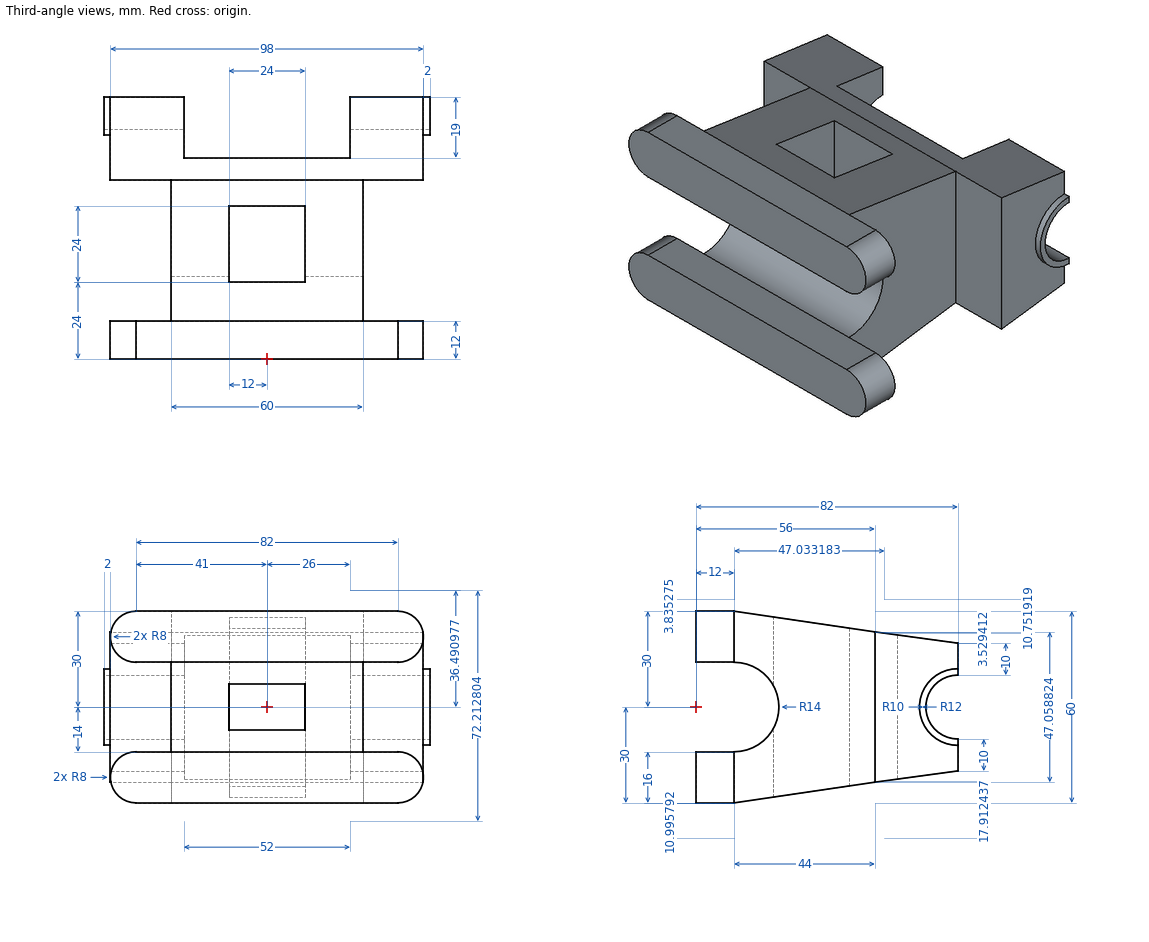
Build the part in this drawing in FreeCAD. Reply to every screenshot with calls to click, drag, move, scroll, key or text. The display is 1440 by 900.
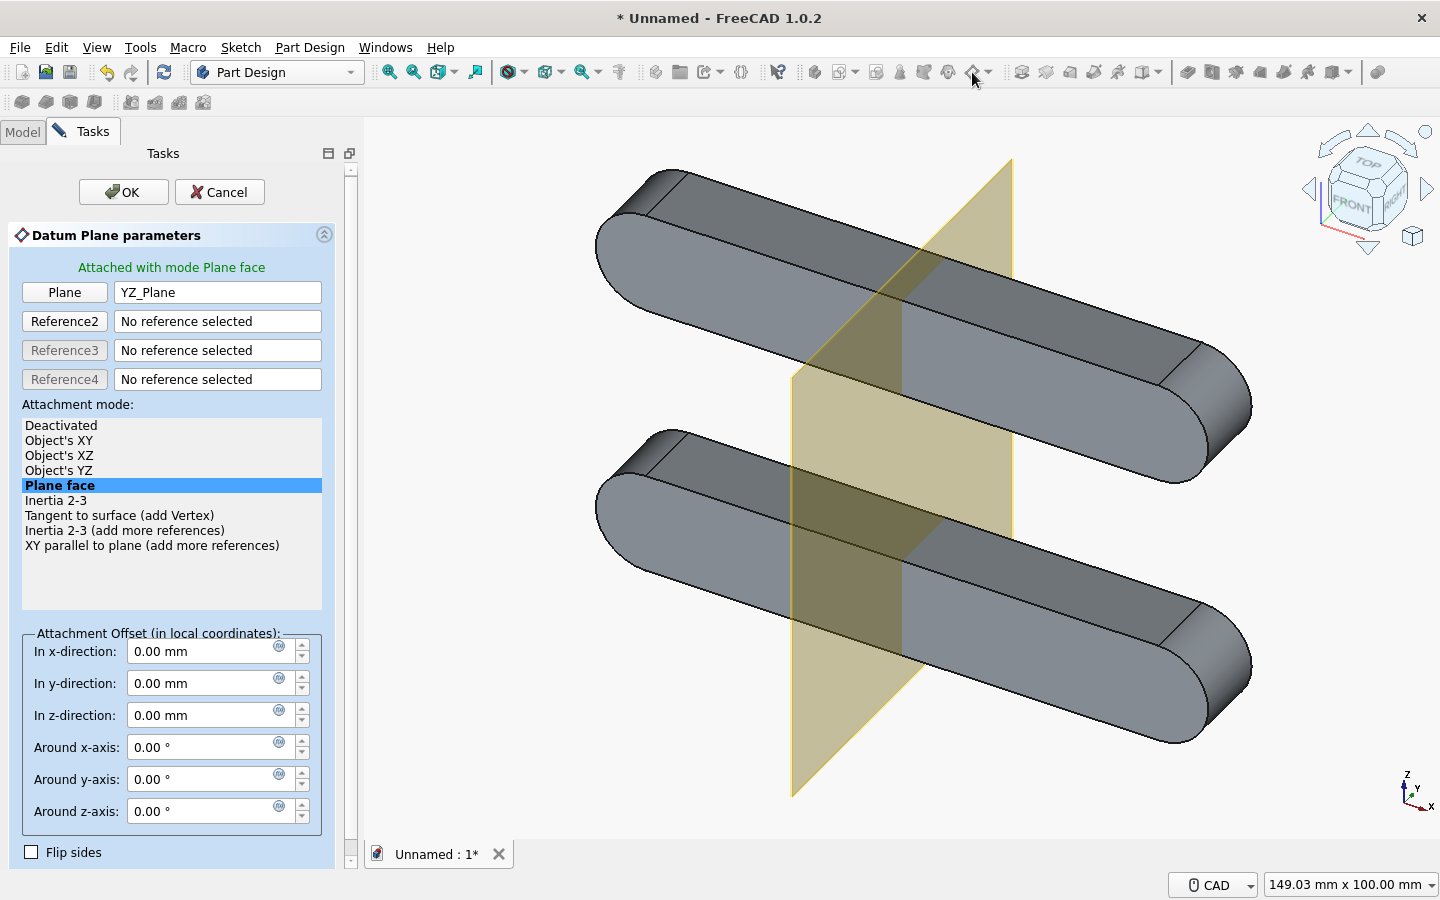
triple_click(210, 715)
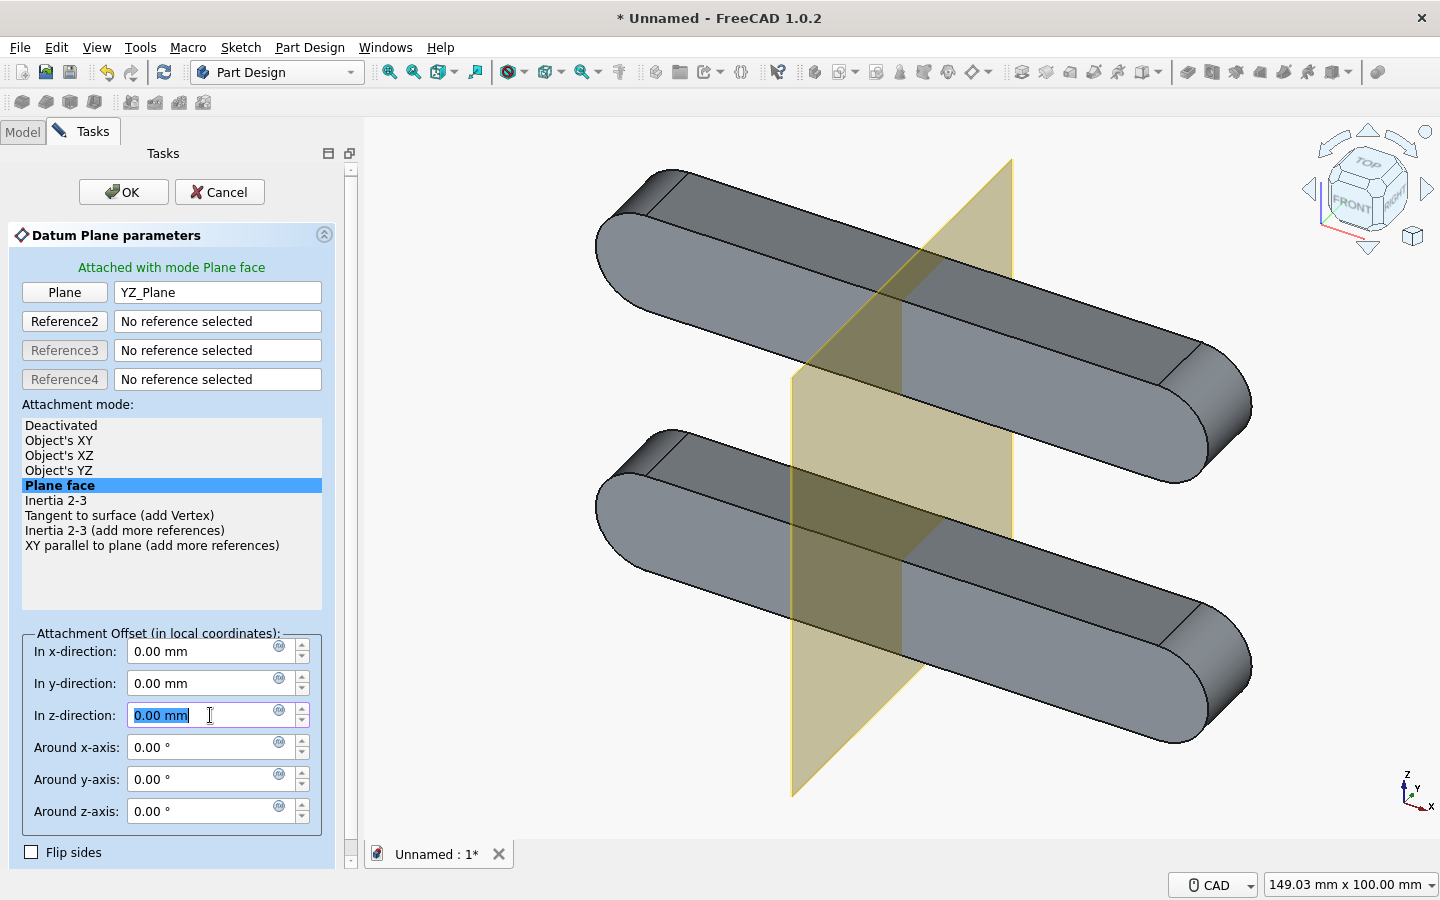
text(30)
key(Tab)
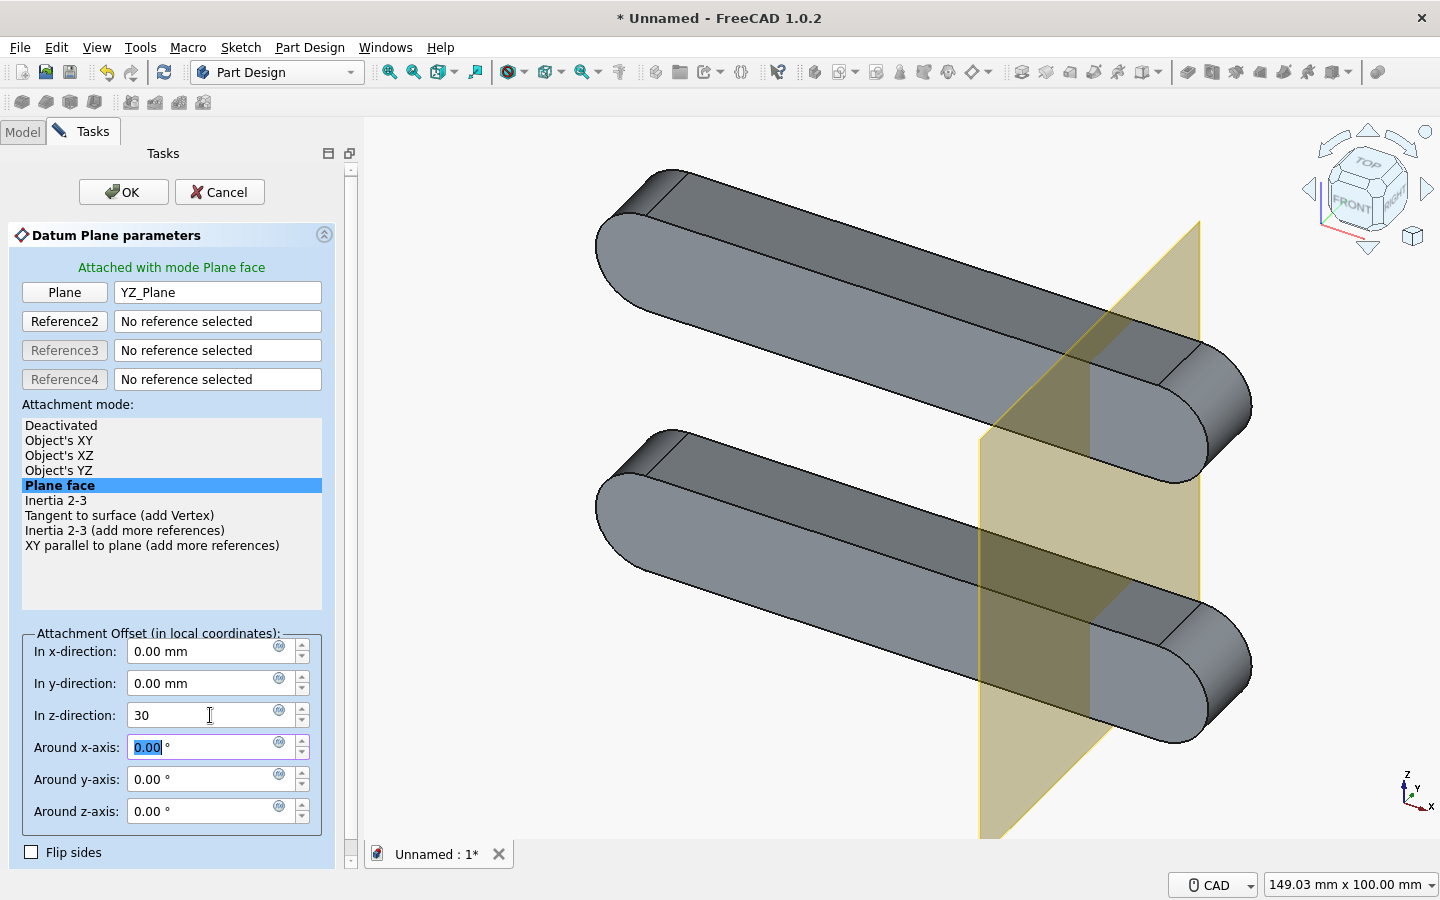
click(124, 192)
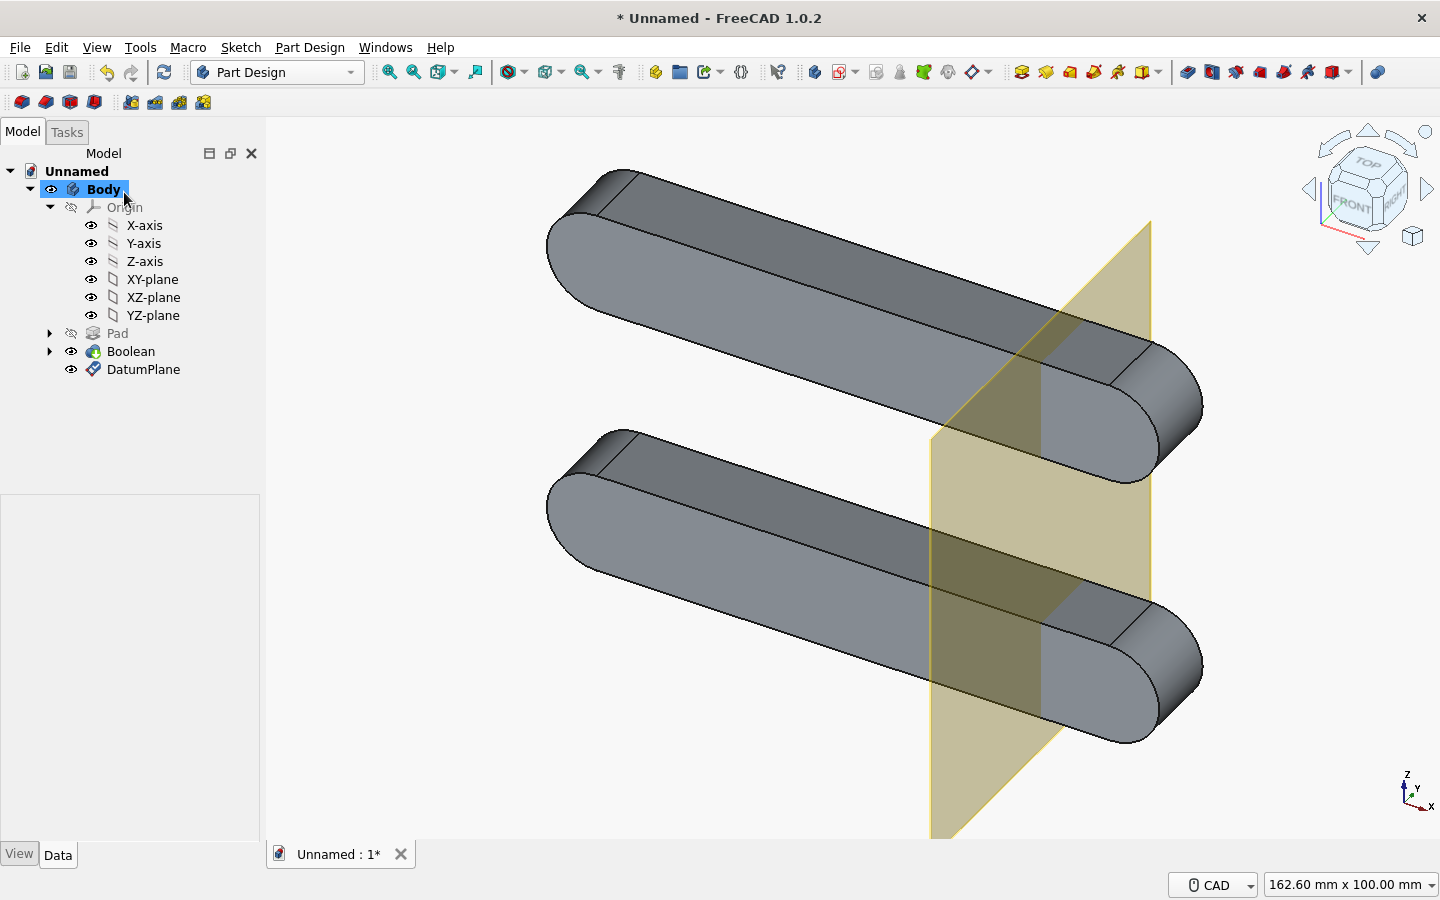
click(116, 369)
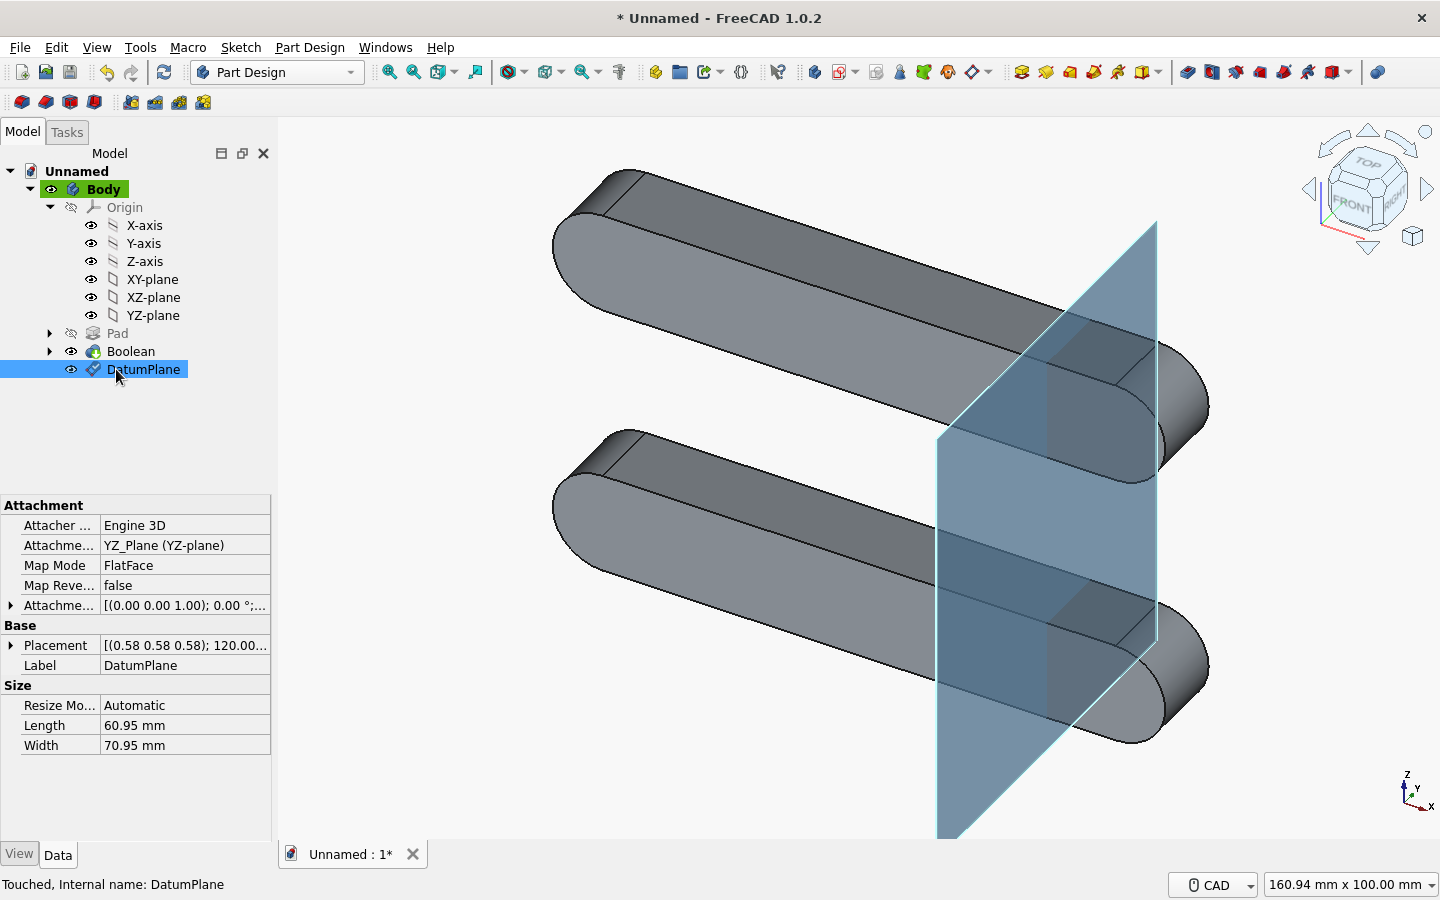
click(840, 72)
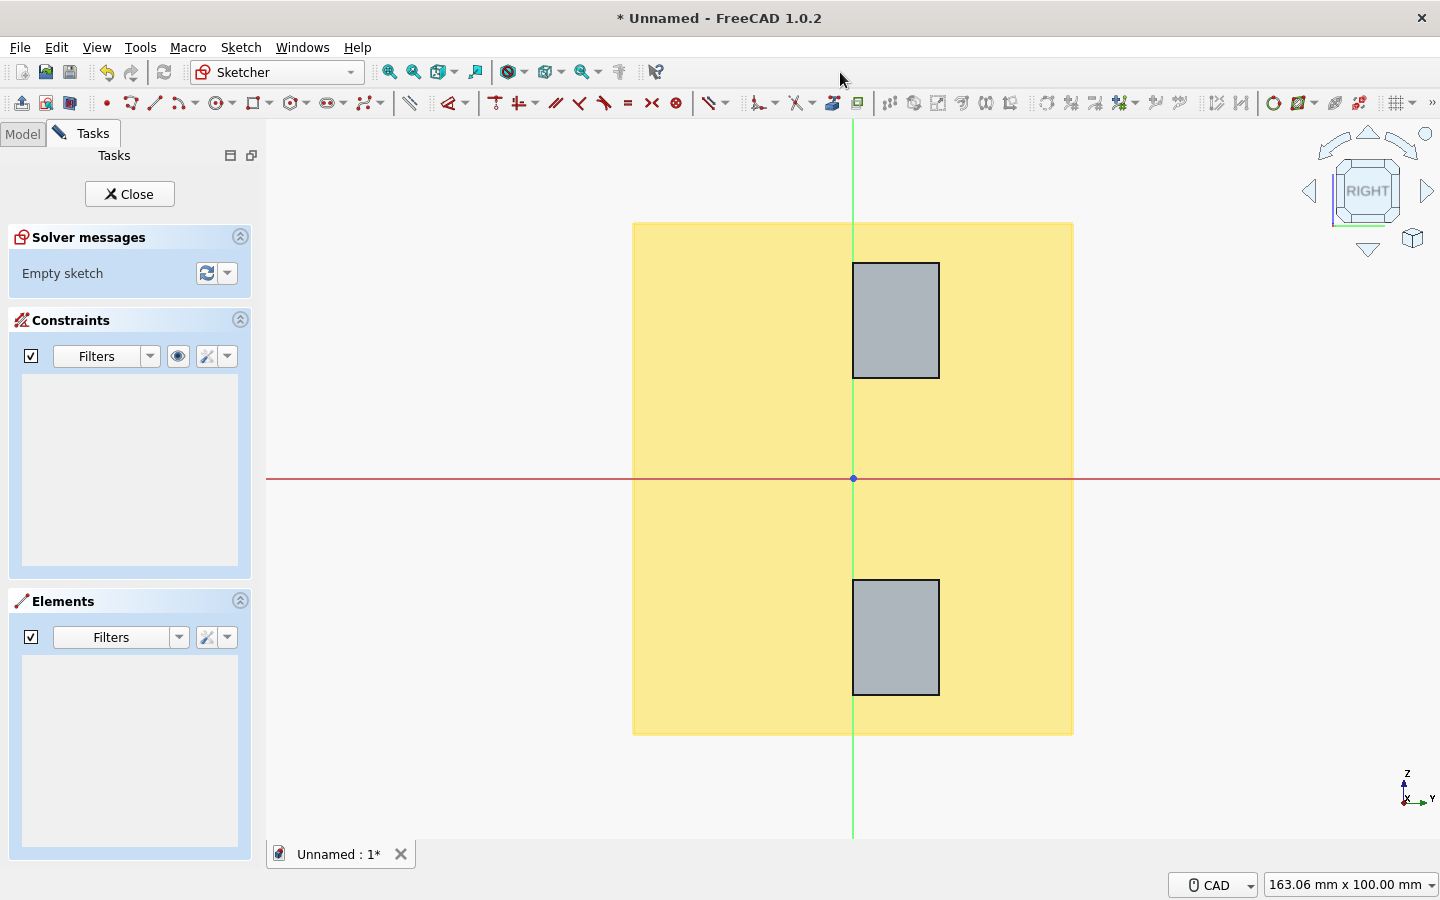
click(70, 104)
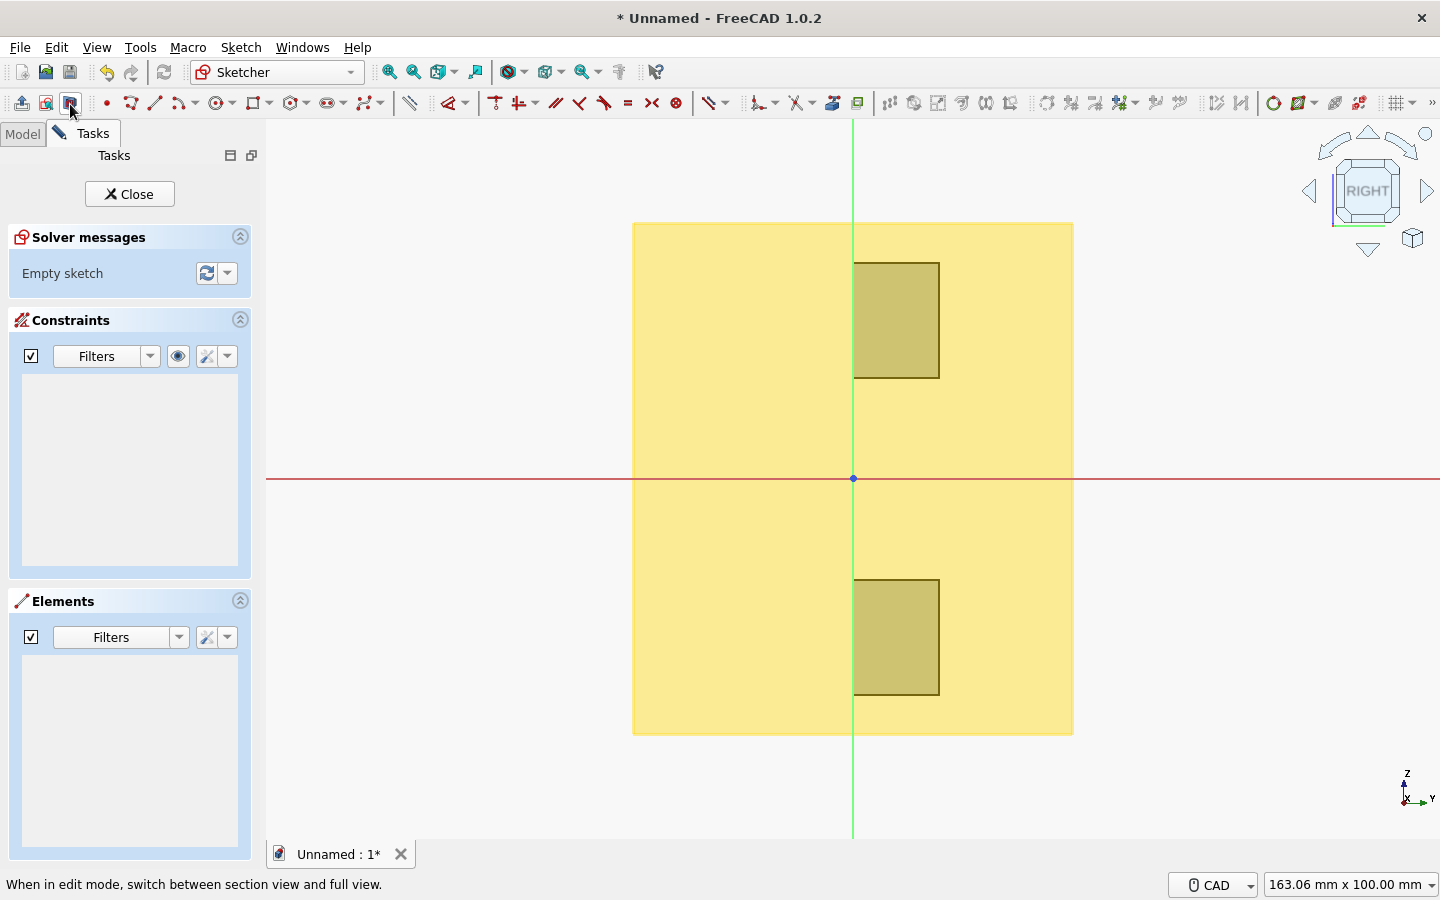
scroll(294, 479, down, 1)